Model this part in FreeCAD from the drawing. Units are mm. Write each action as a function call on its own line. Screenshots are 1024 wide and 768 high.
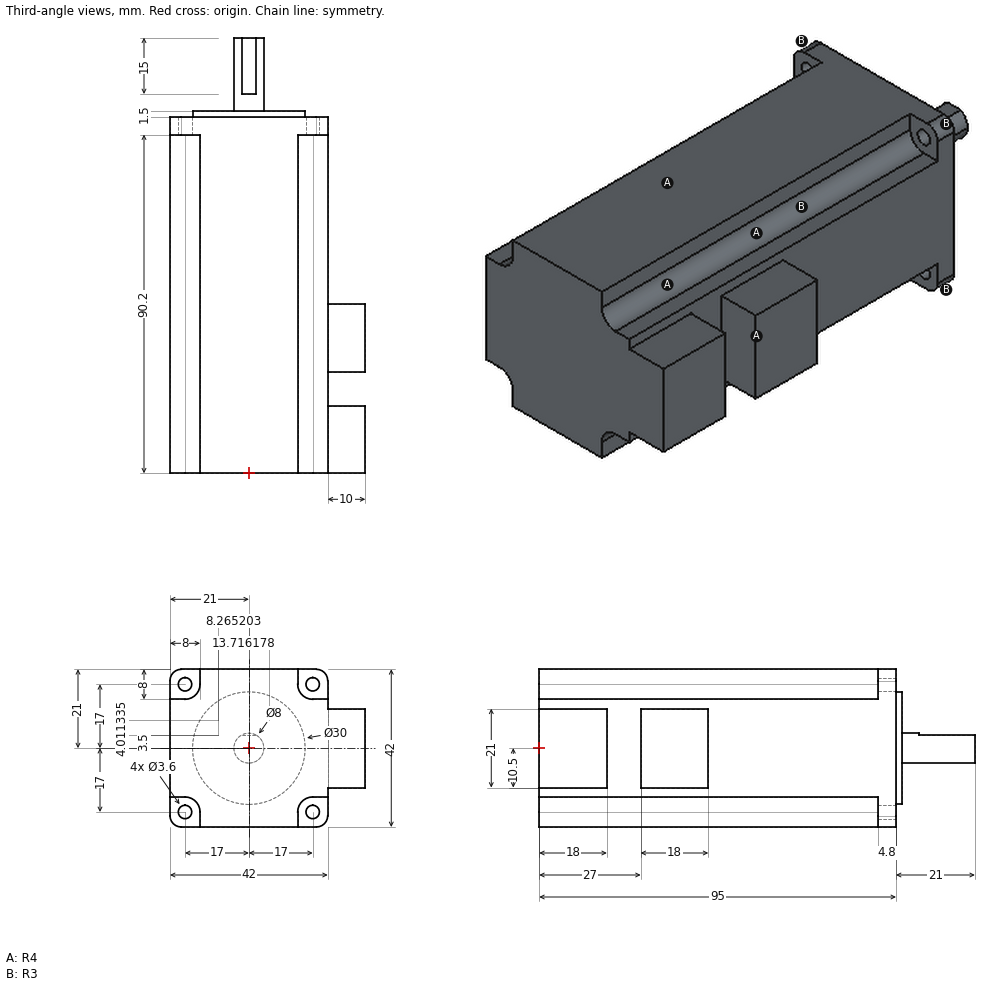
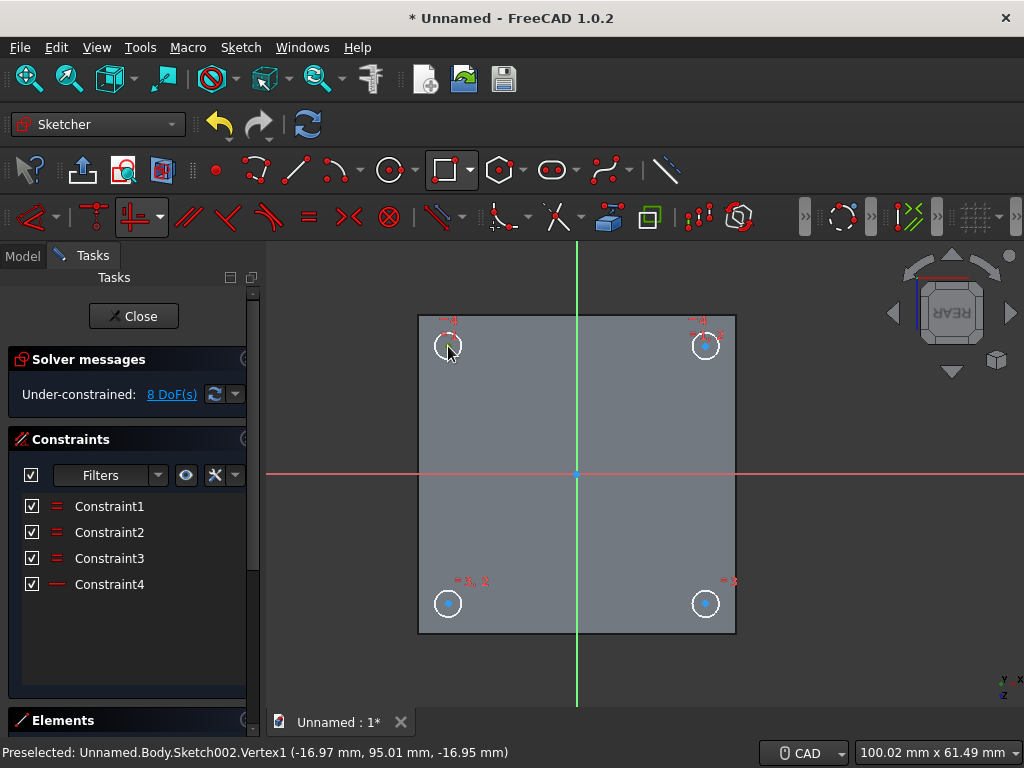
click(448, 604)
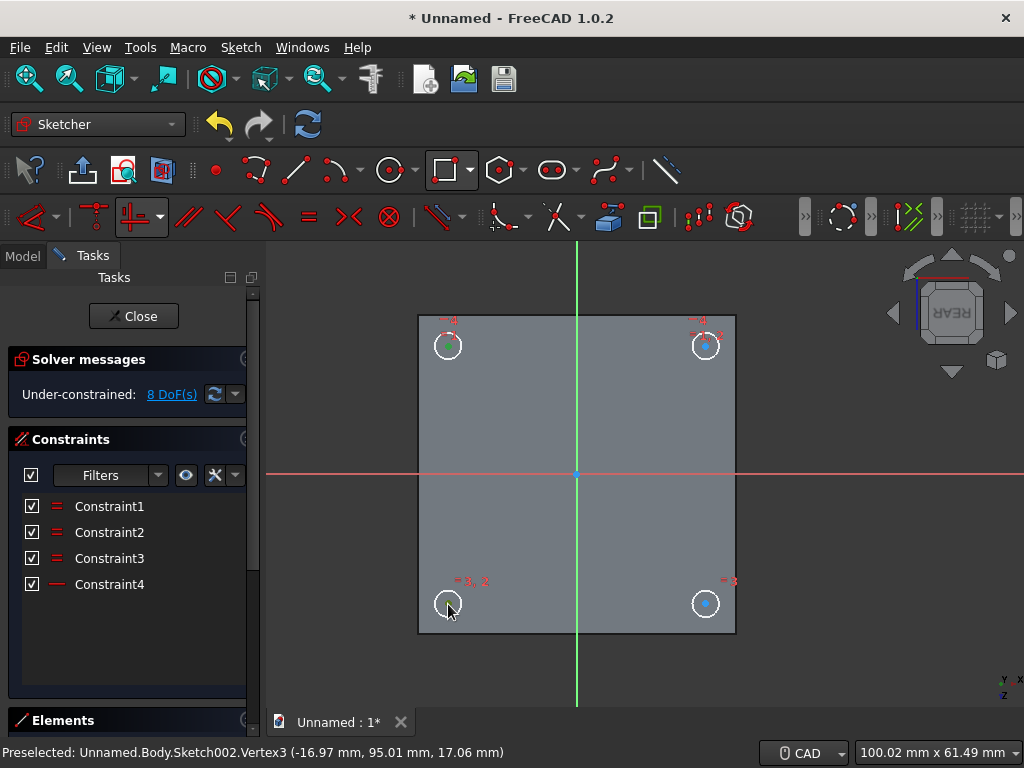
click(162, 218)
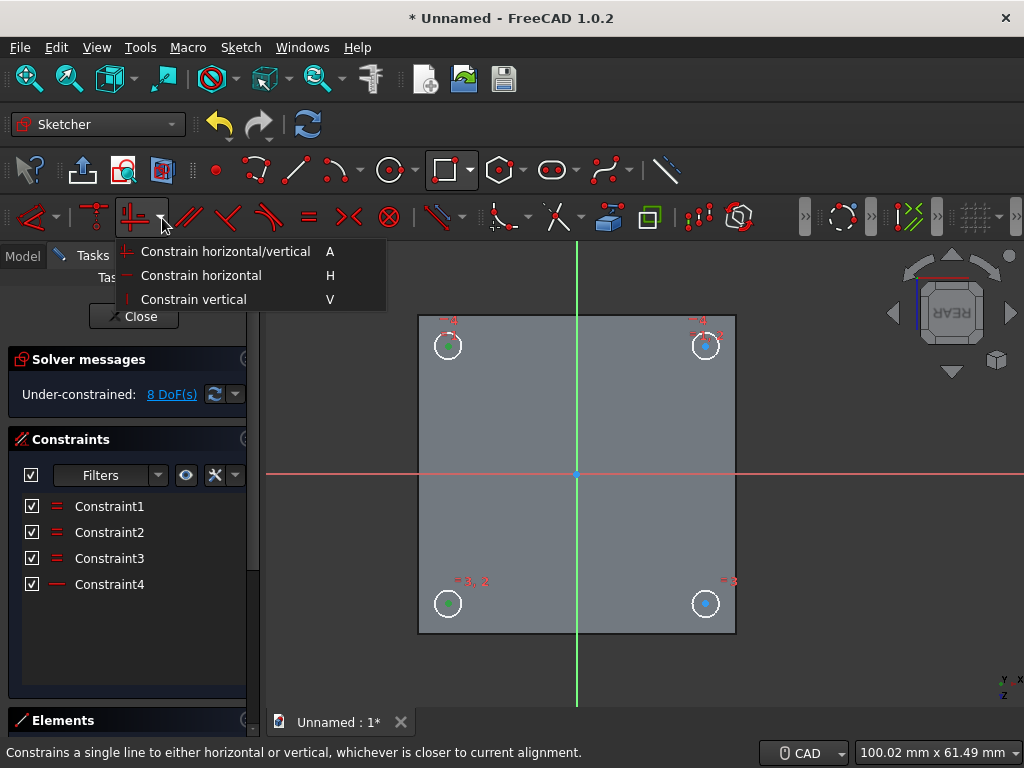
click(251, 299)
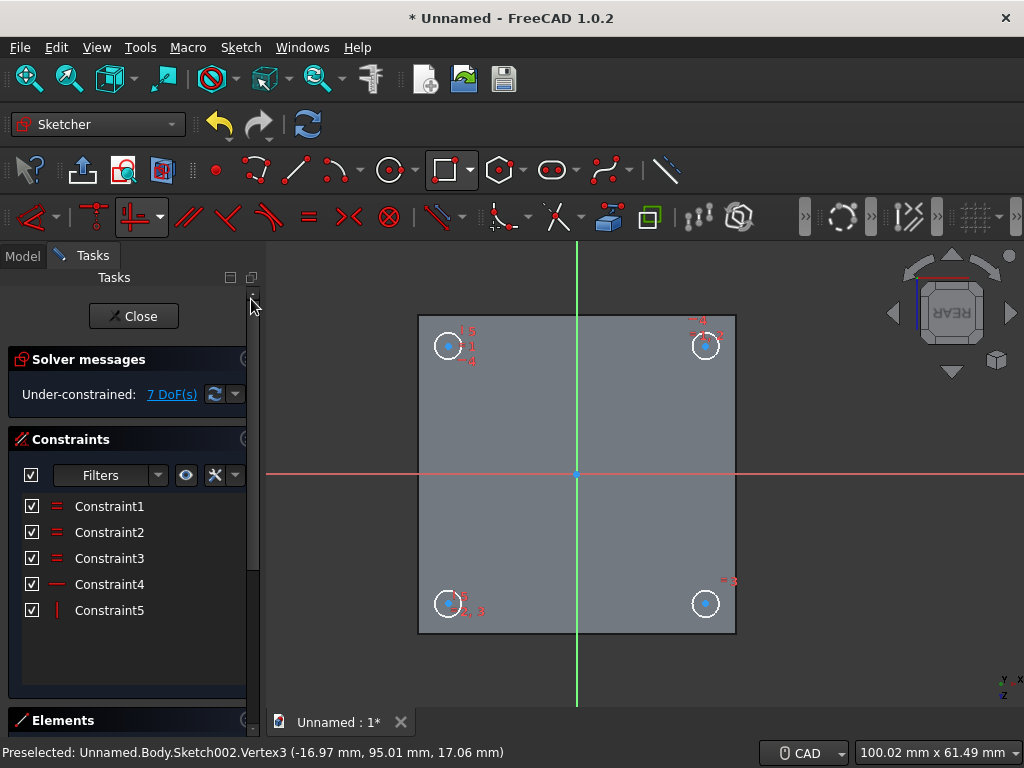
click(706, 346)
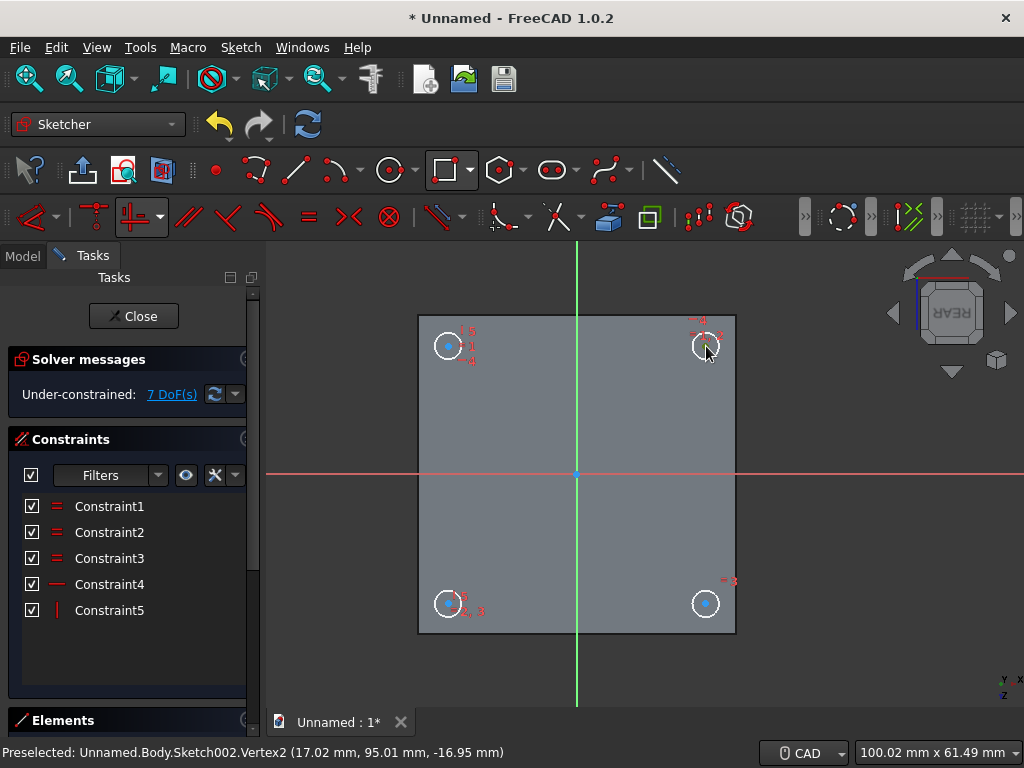
click(706, 604)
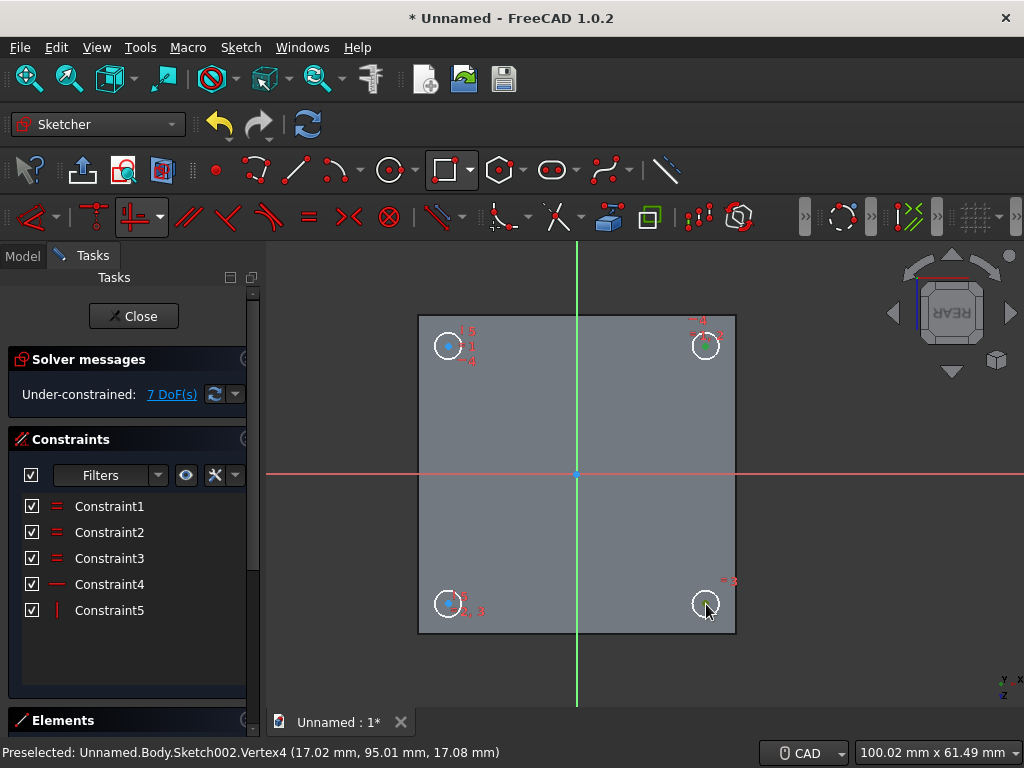
click(162, 218)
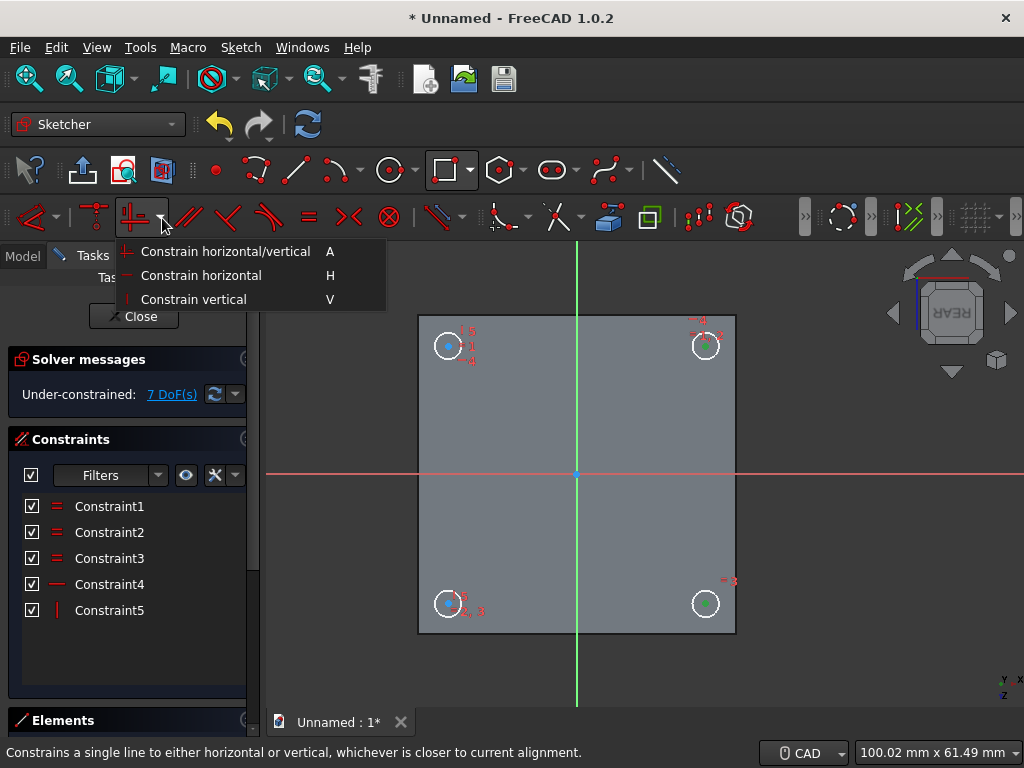
click(251, 299)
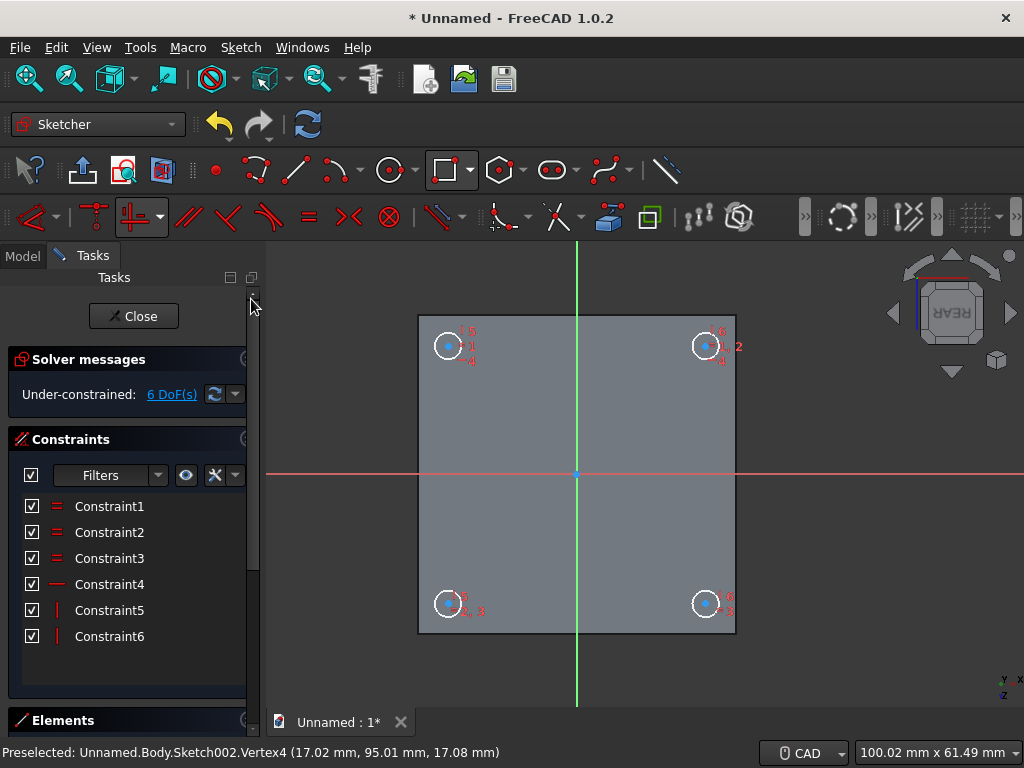
click(448, 604)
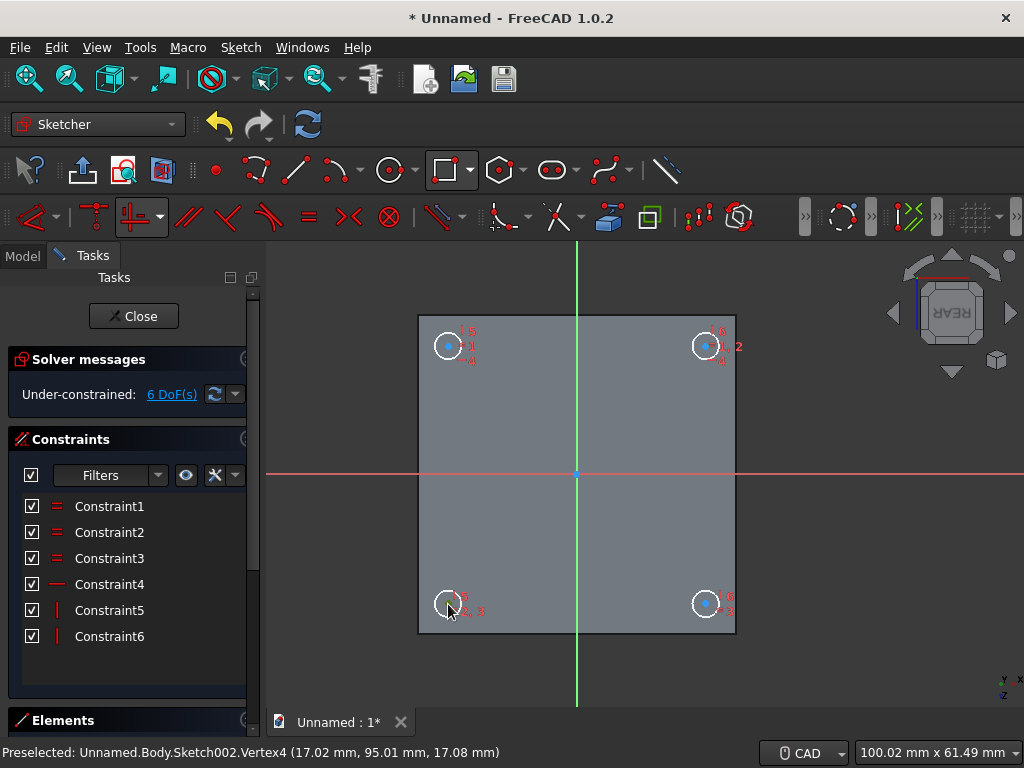
click(706, 604)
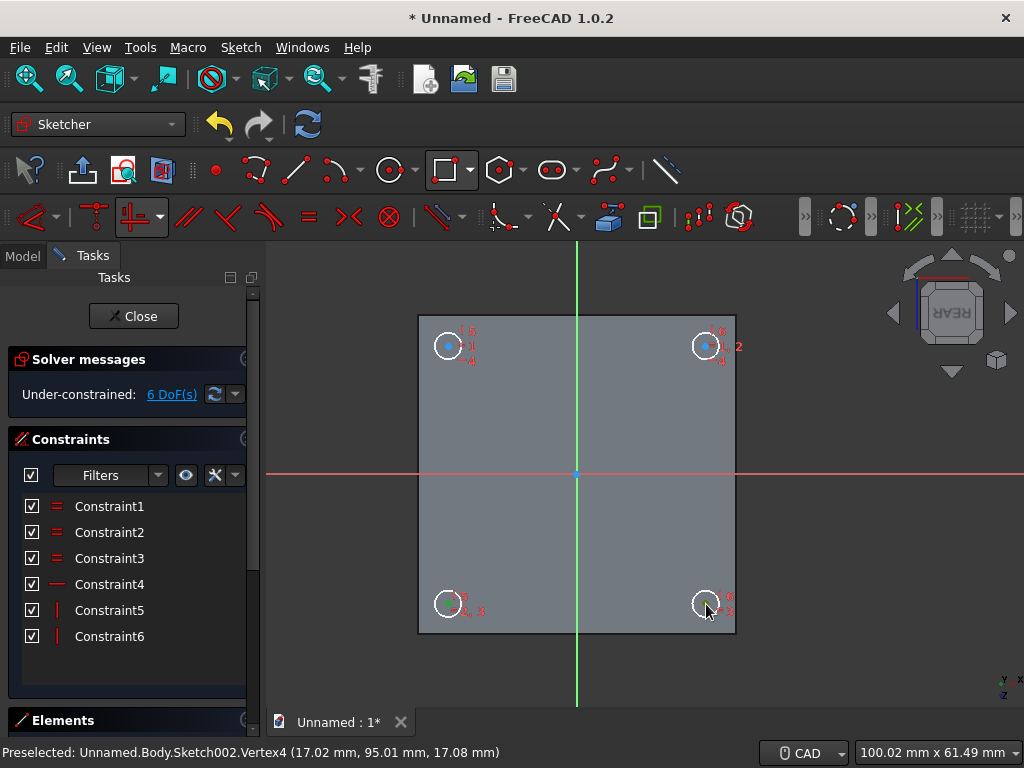
key(h)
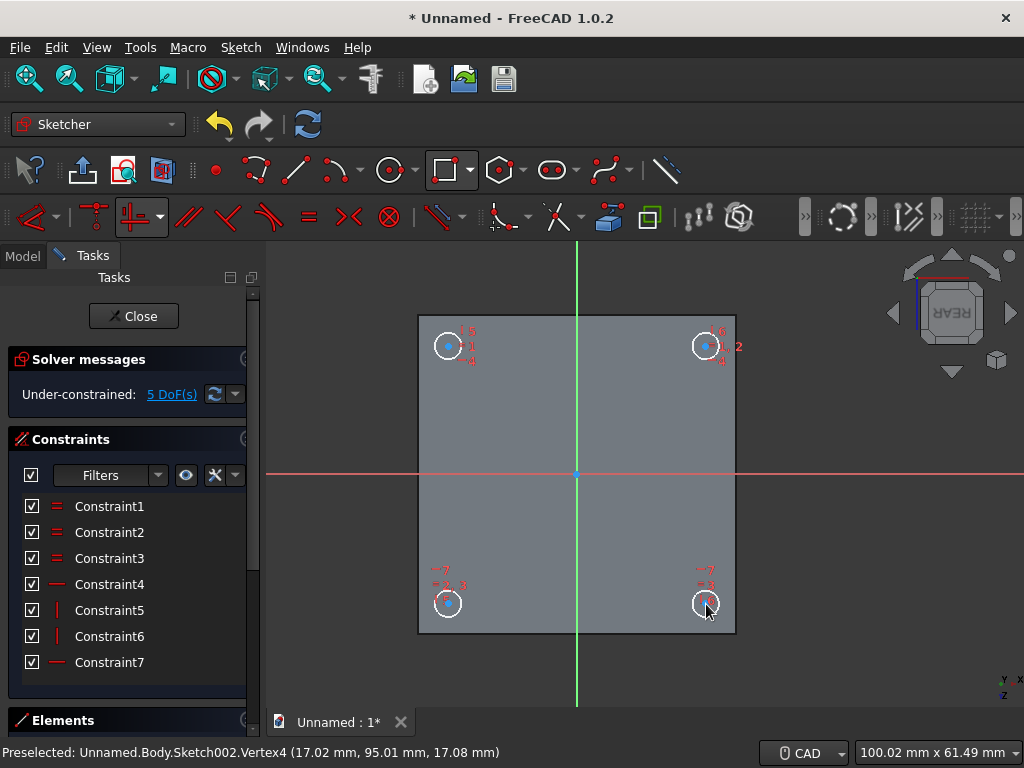
click(32, 218)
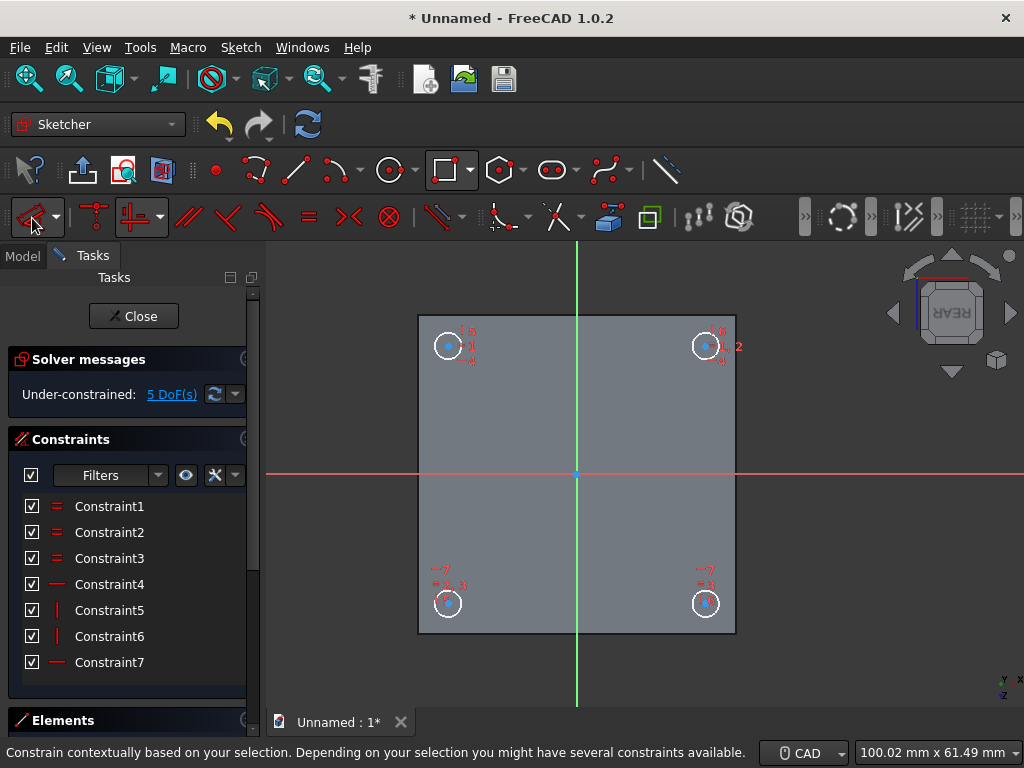
scroll(457, 337, up, 2)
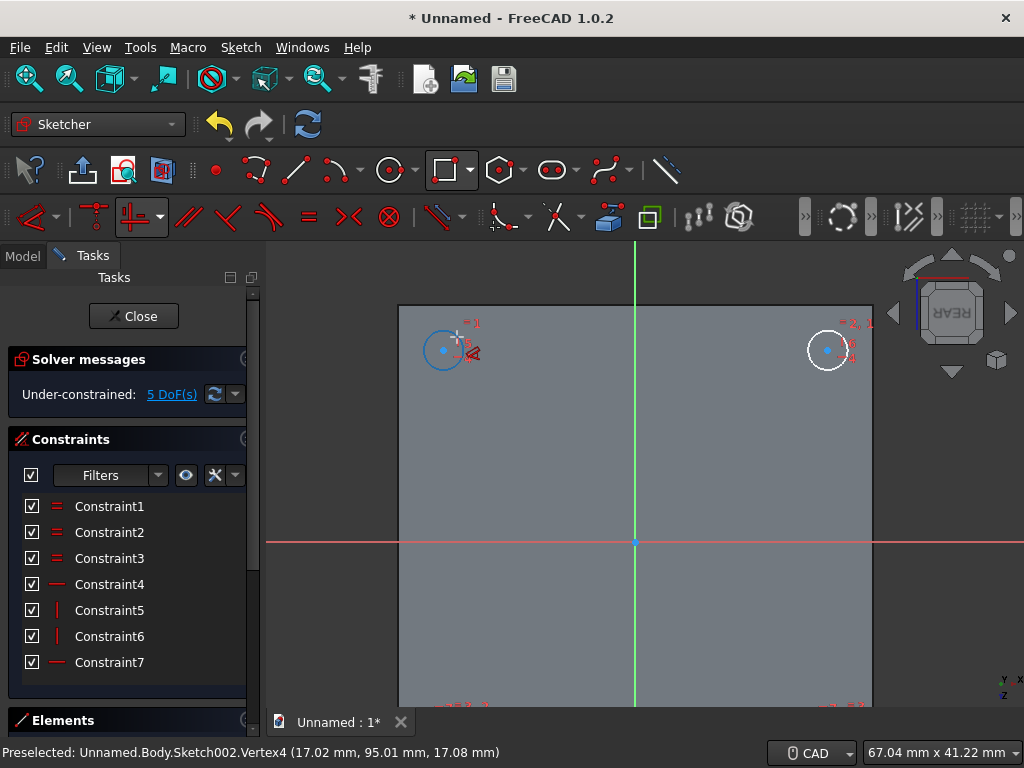
click(457, 336)
click(479, 313)